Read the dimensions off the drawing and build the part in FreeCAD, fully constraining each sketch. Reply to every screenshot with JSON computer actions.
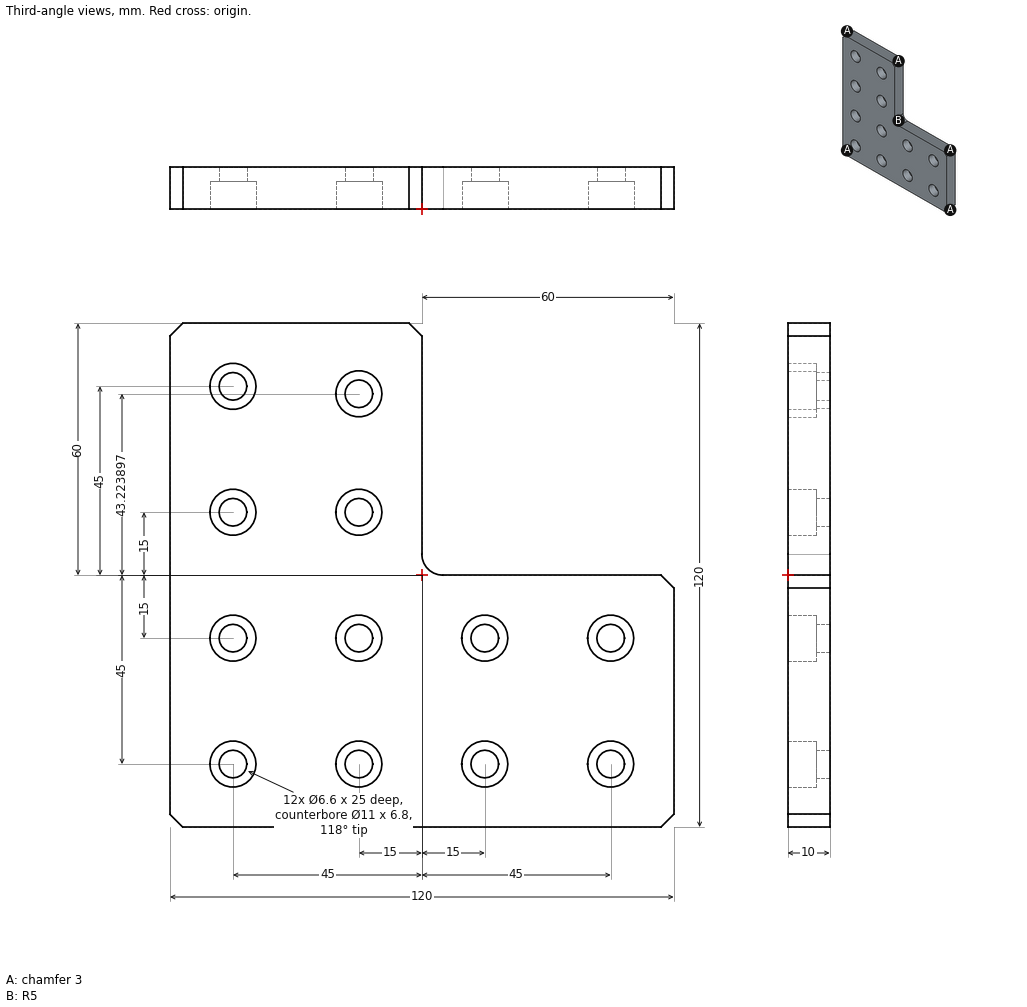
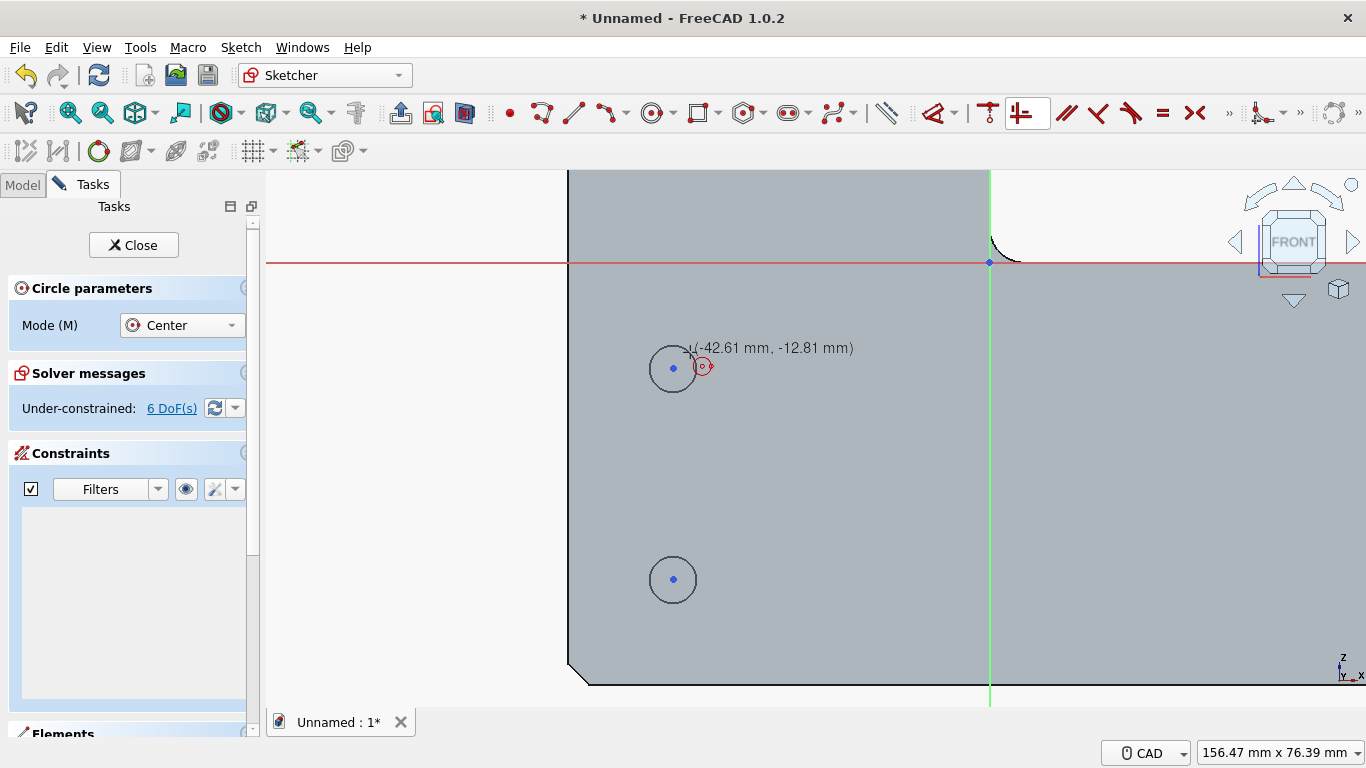
{"action": "left_click", "coordinate": [884, 579]}
{"action": "left_click", "coordinate": [901, 563]}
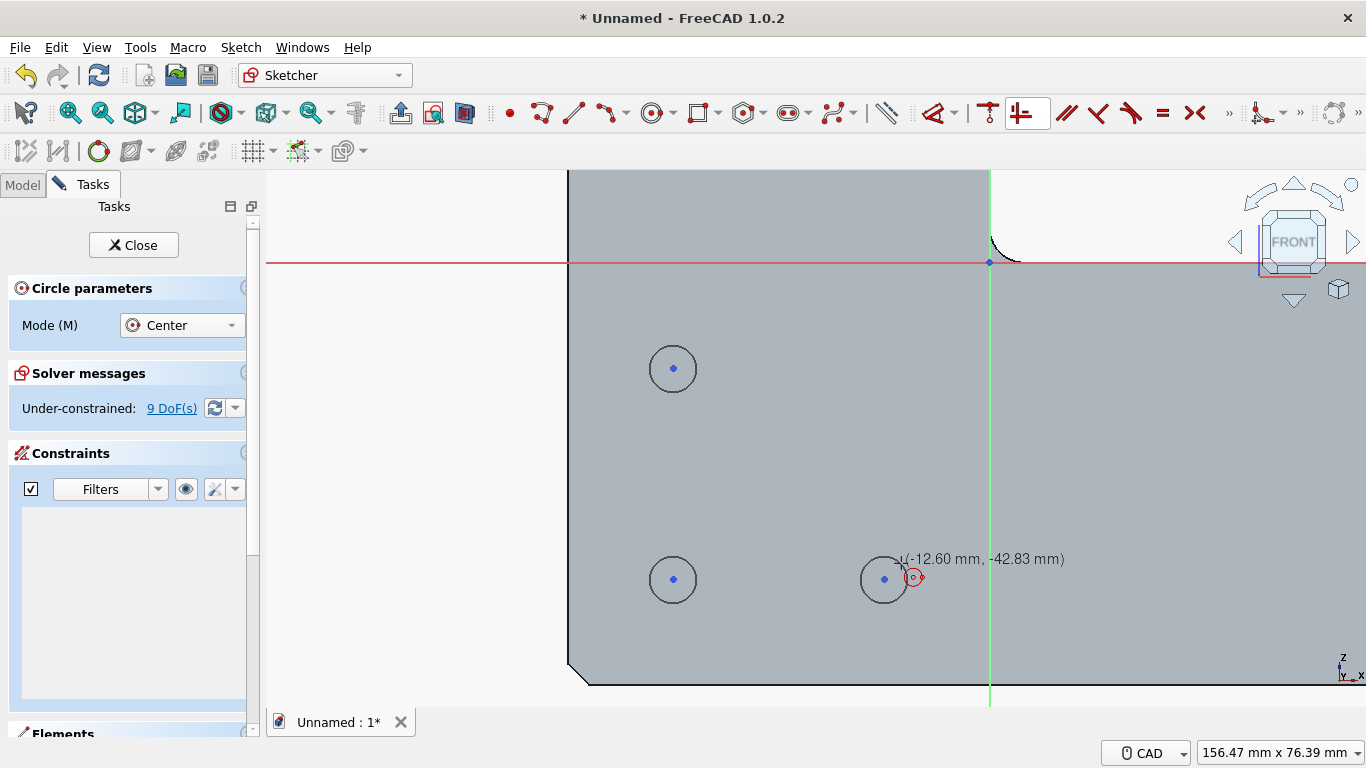
{"action": "left_click", "coordinate": [884, 368]}
{"action": "left_click", "coordinate": [901, 352]}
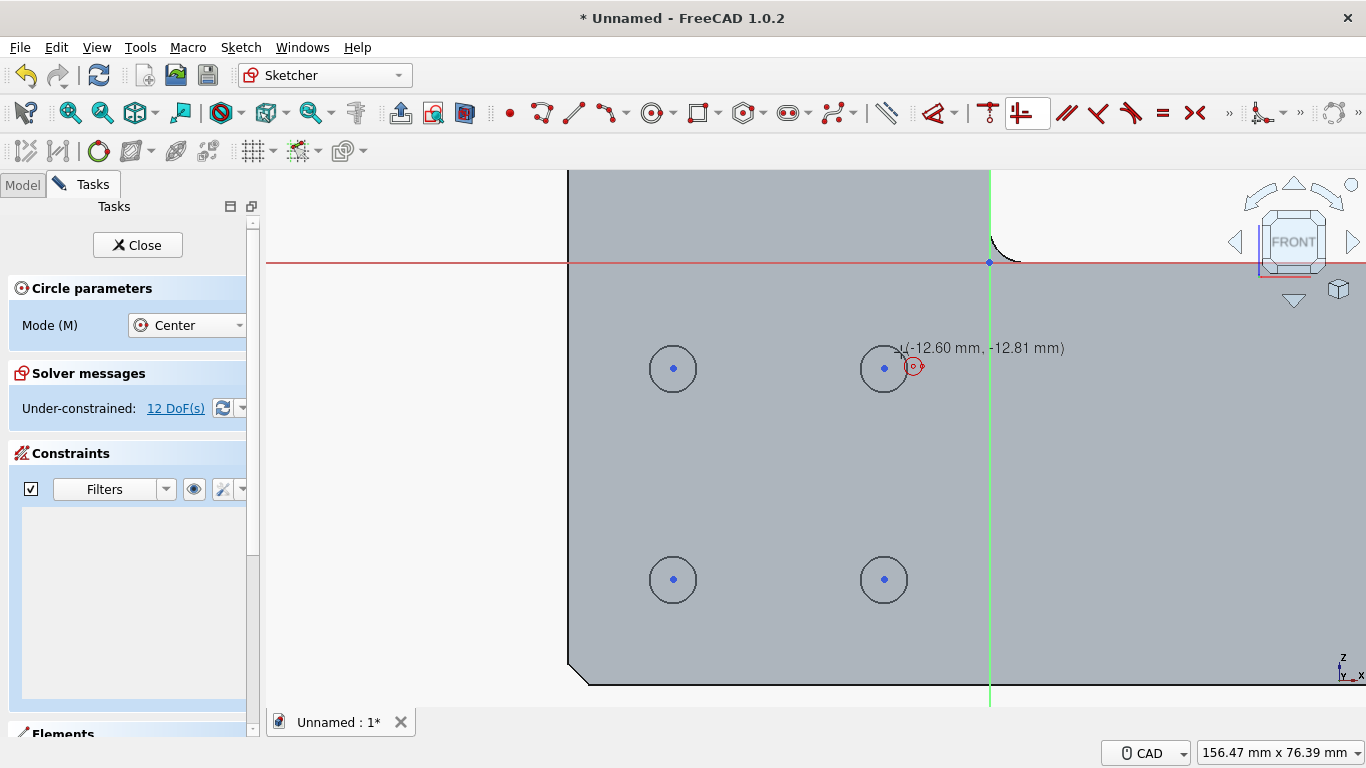
{"action": "scroll", "coordinate": [453, 652], "scroll_direction": "down", "scroll_amount": 3}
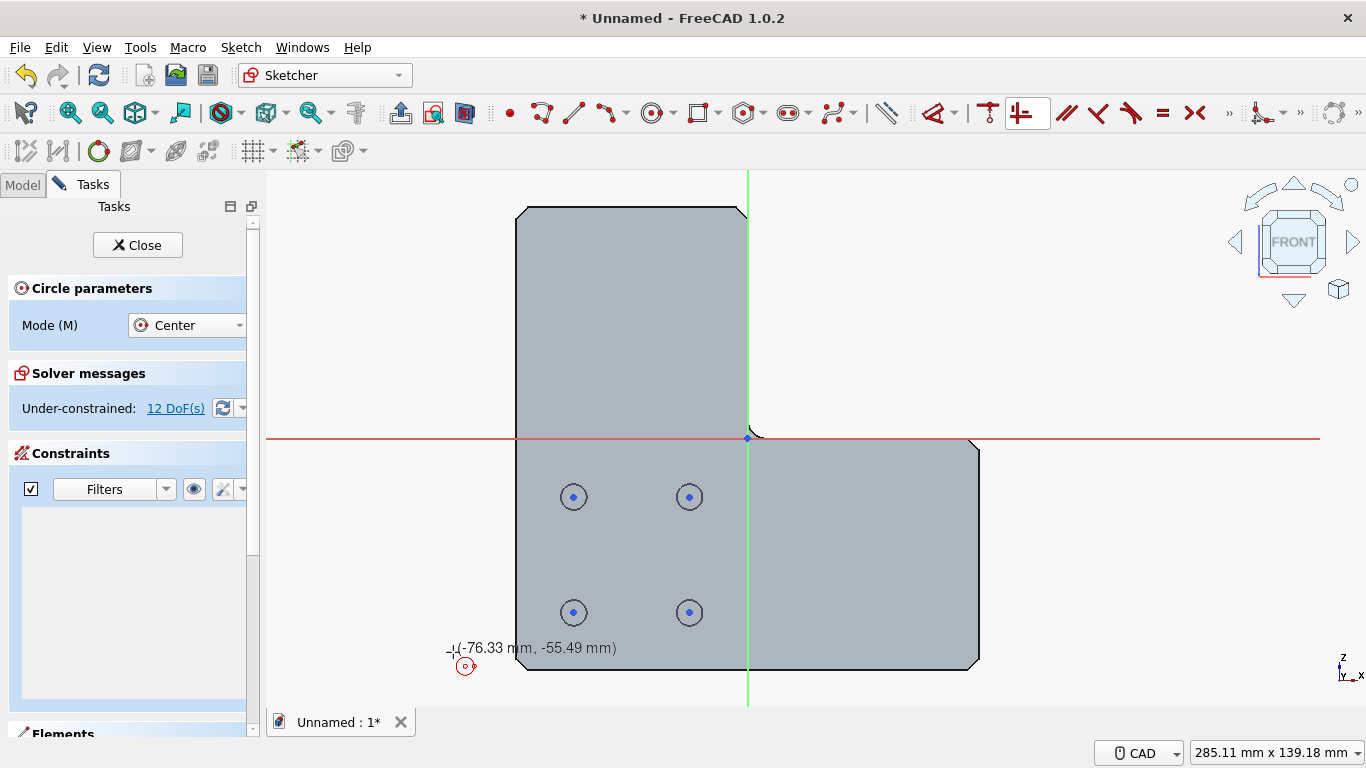
{"action": "scroll", "coordinate": [921, 612], "scroll_direction": "up", "scroll_amount": 3}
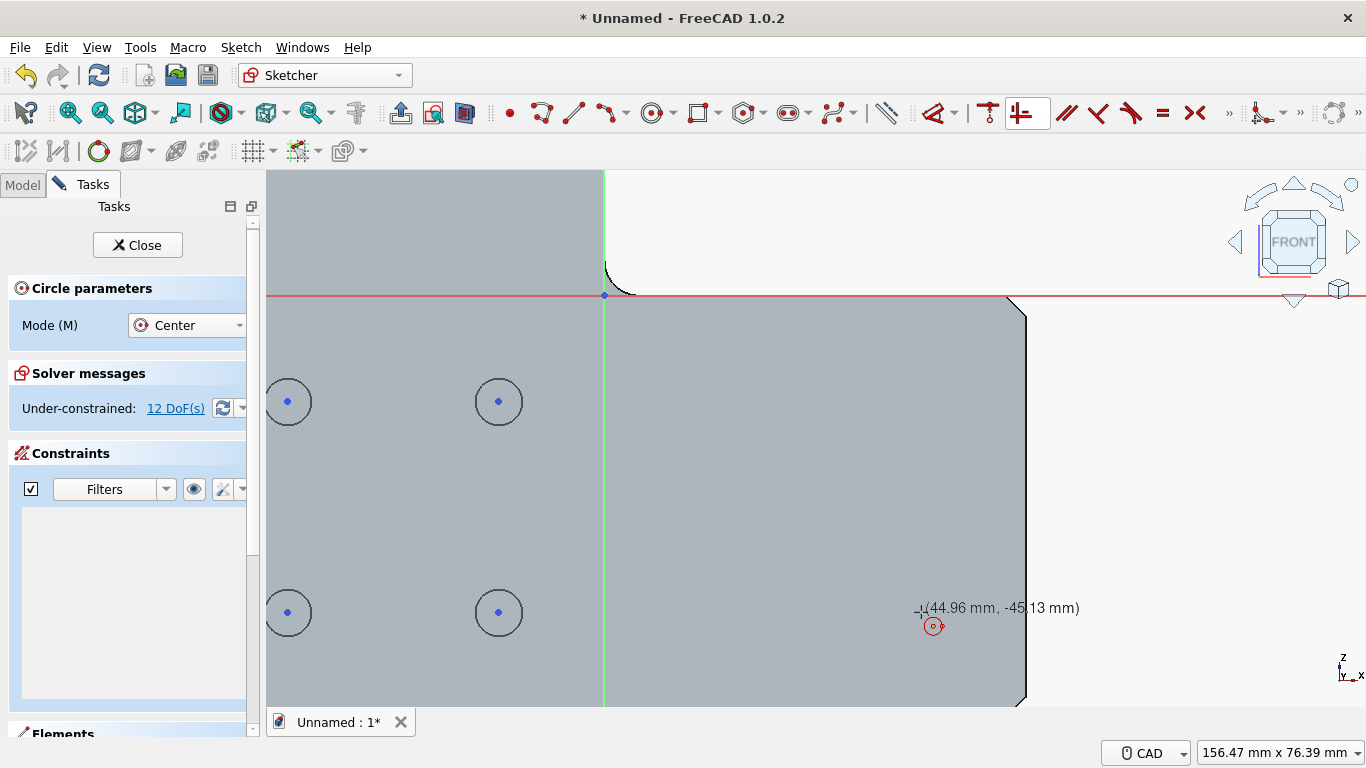
{"action": "left_click", "coordinate": [921, 612]}
{"action": "left_click", "coordinate": [937, 596]}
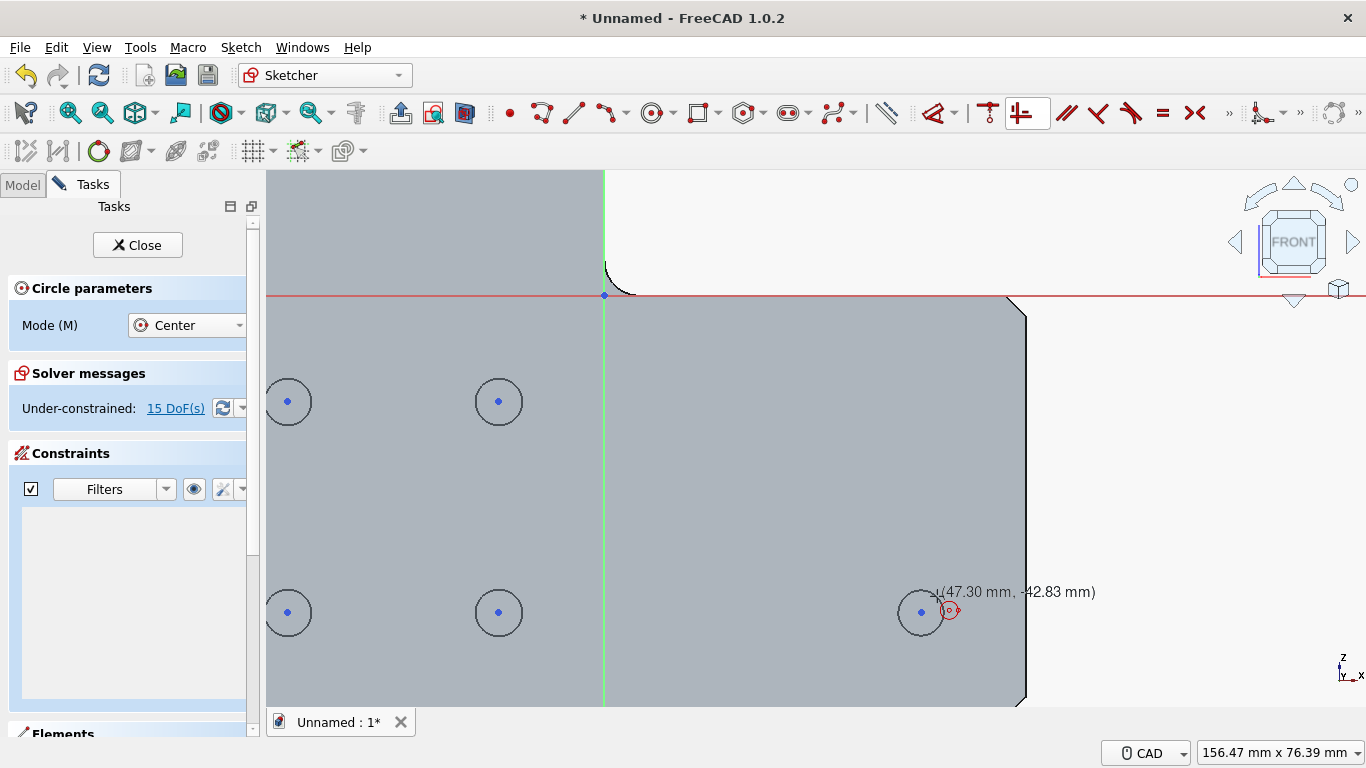
{"action": "left_click", "coordinate": [921, 401]}
{"action": "left_click", "coordinate": [937, 385]}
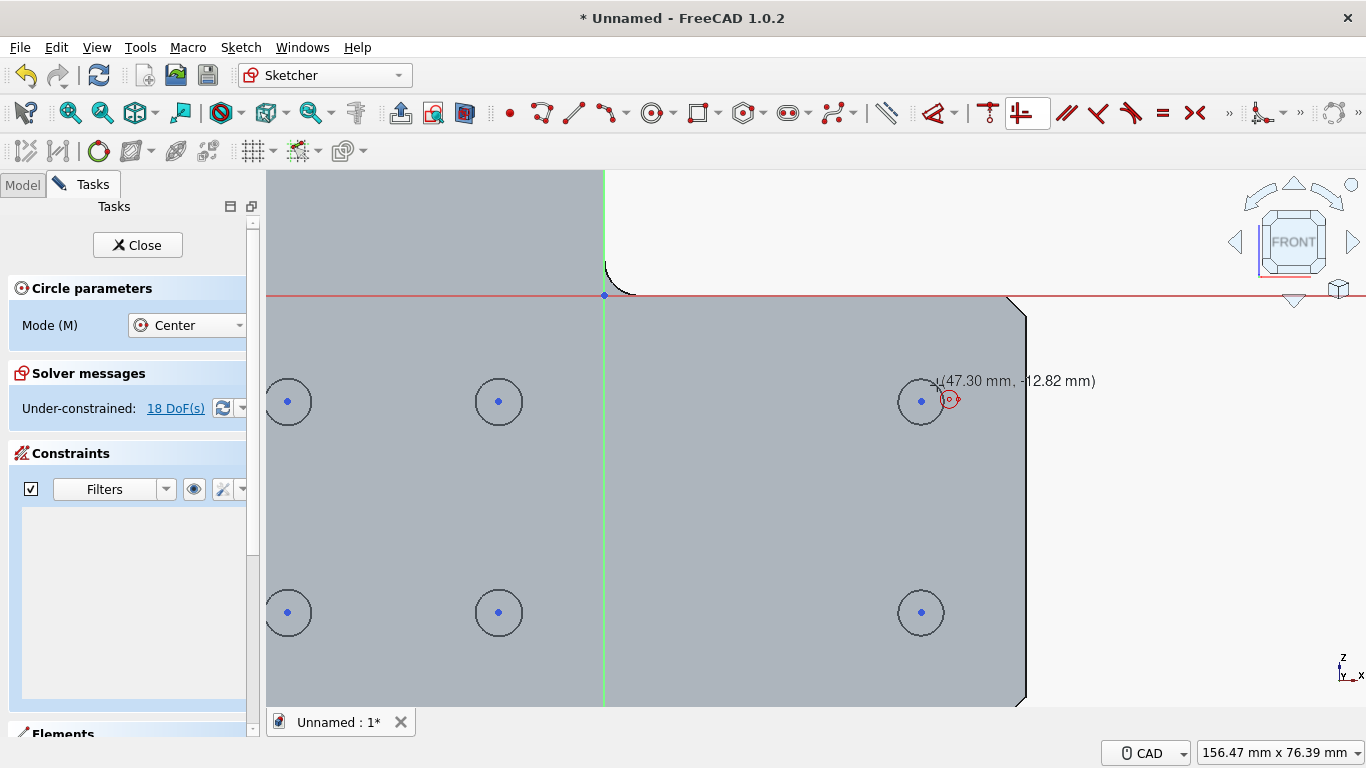
{"action": "scroll", "coordinate": [921, 612], "scroll_direction": "down", "scroll_amount": 3}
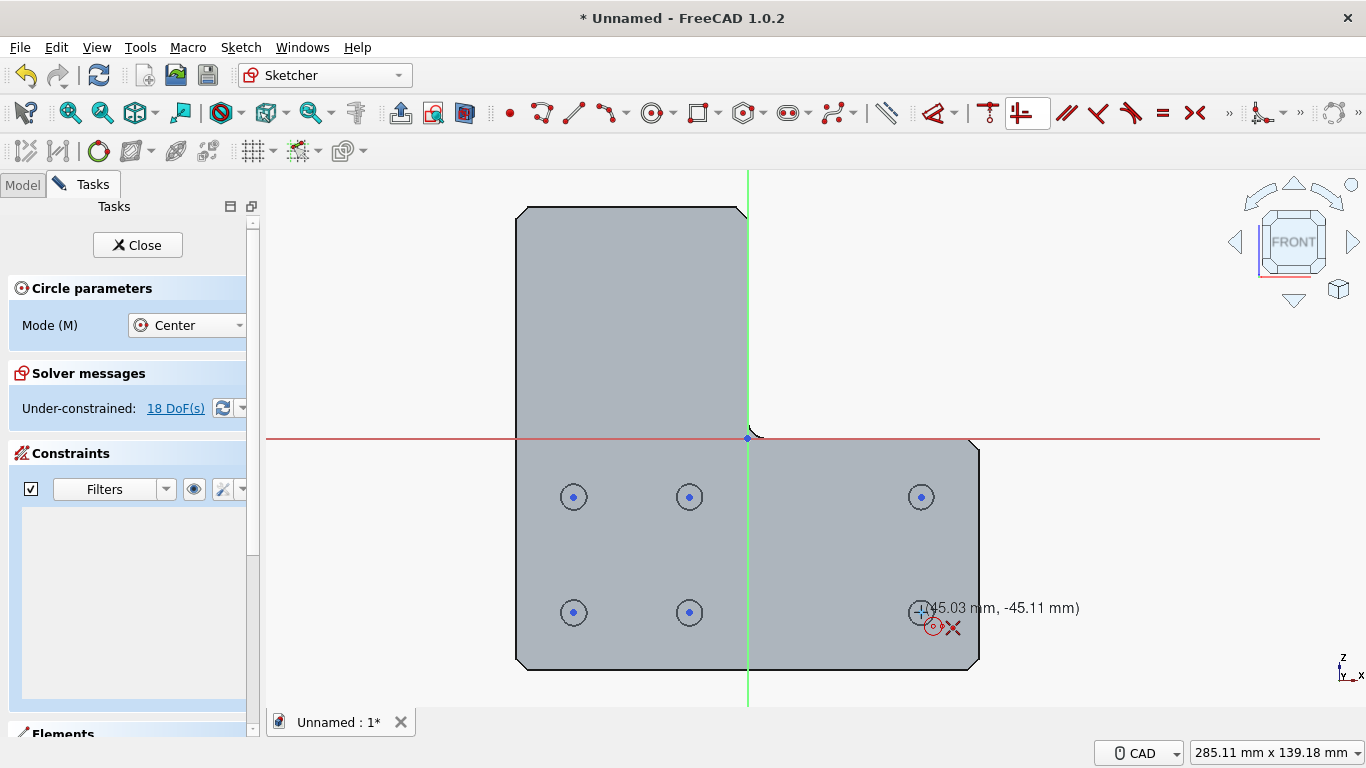
{"action": "scroll", "coordinate": [574, 381], "scroll_direction": "up", "scroll_amount": 3}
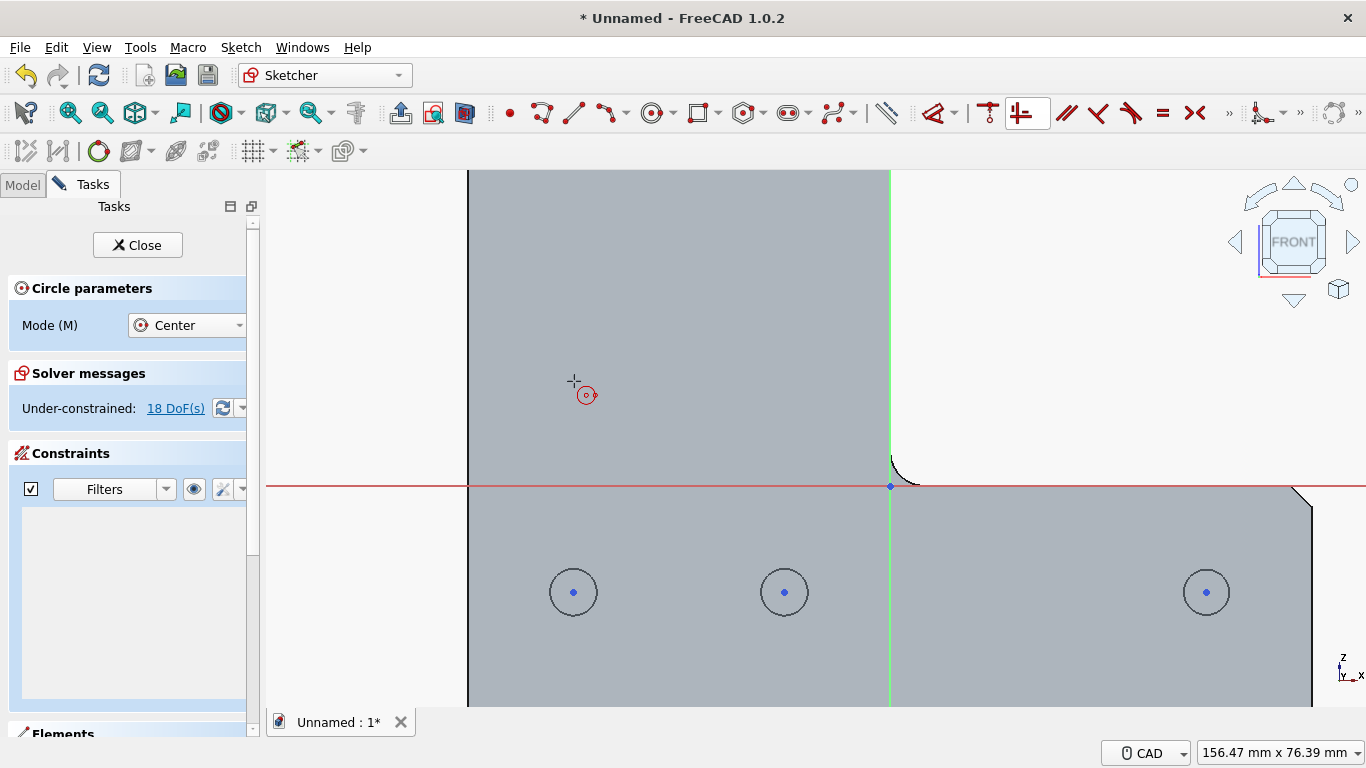
{"action": "left_click", "coordinate": [574, 381]}
{"action": "left_click", "coordinate": [590, 364]}